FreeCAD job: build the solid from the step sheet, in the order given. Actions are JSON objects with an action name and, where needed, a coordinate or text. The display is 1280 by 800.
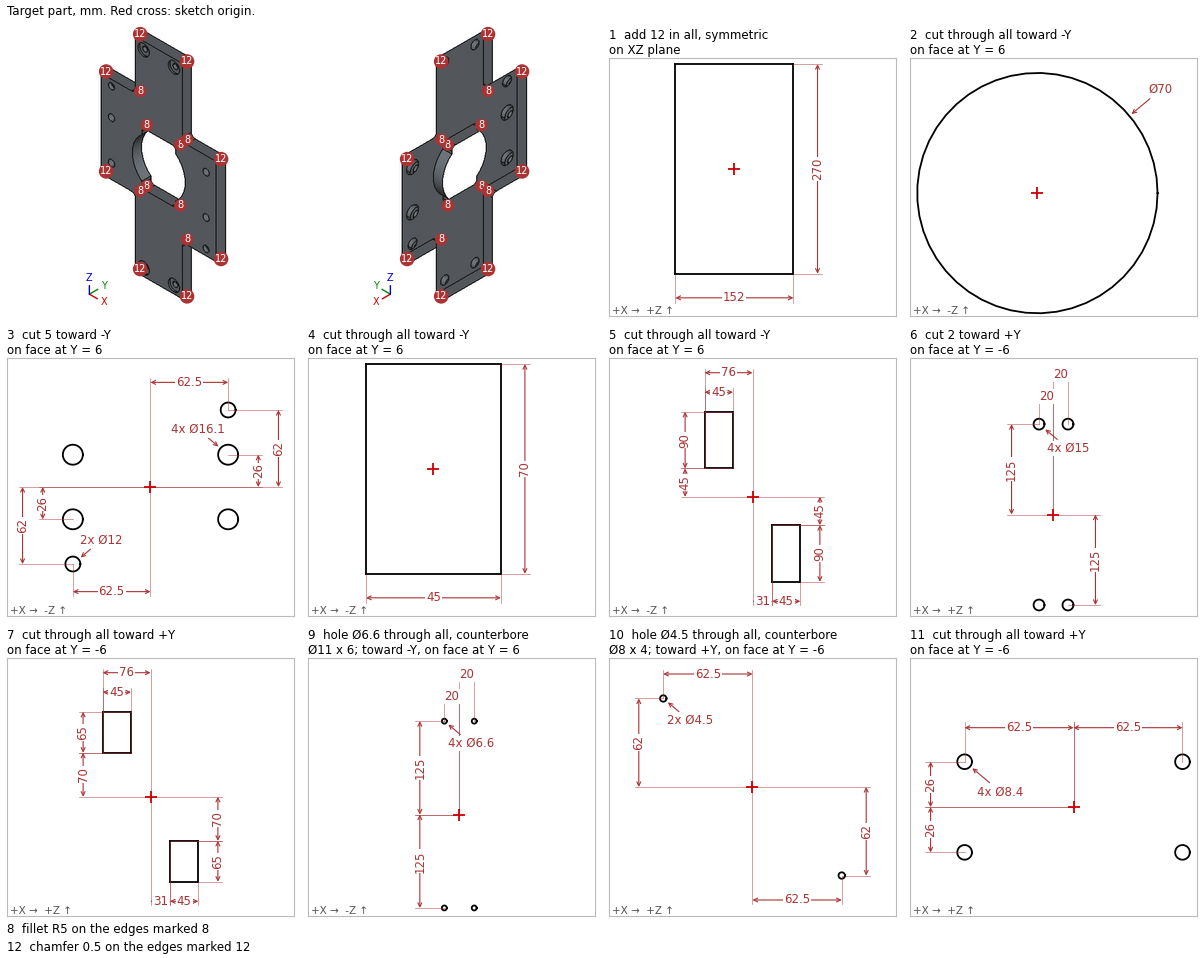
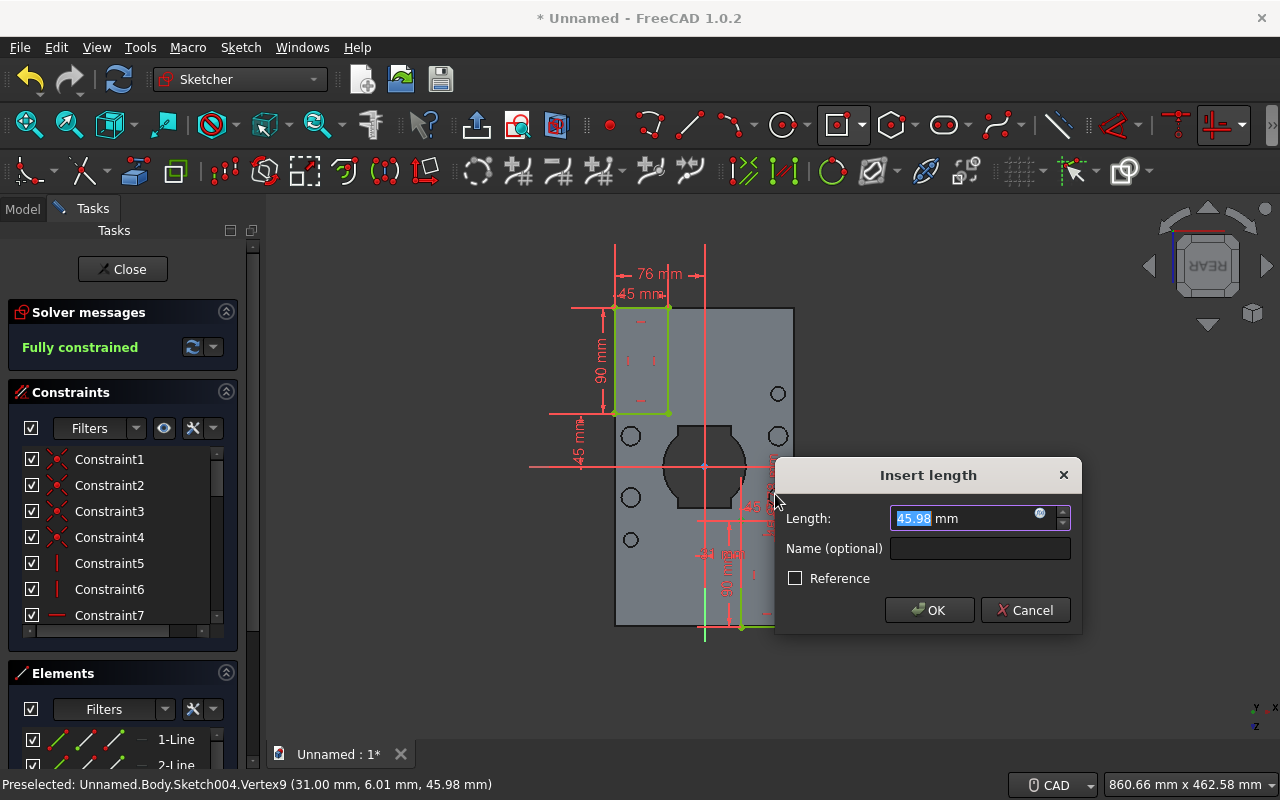
{"action": "type", "text": "45"}
{"action": "key", "text": "Return"}
{"action": "key", "text": "Escape"}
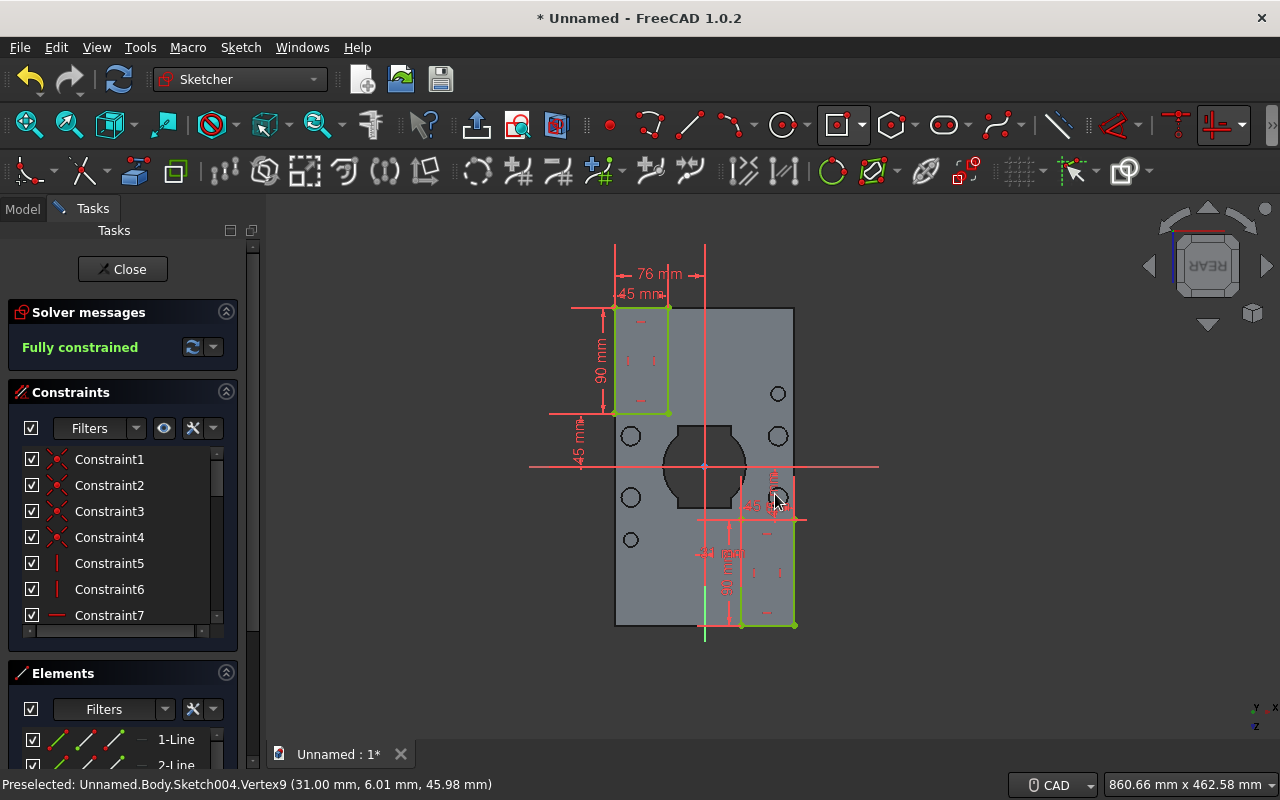
{"action": "left_click", "coordinate": [123, 269]}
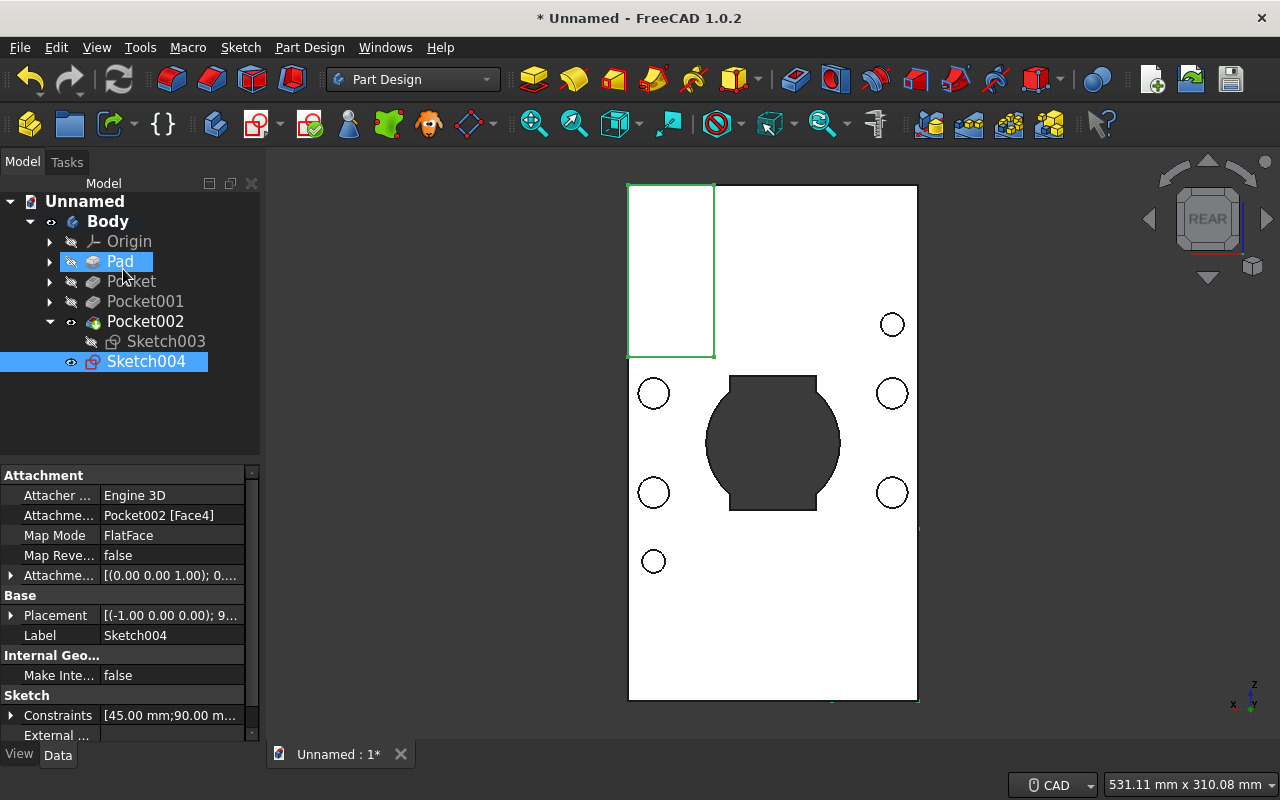
{"action": "left_click", "coordinate": [796, 80]}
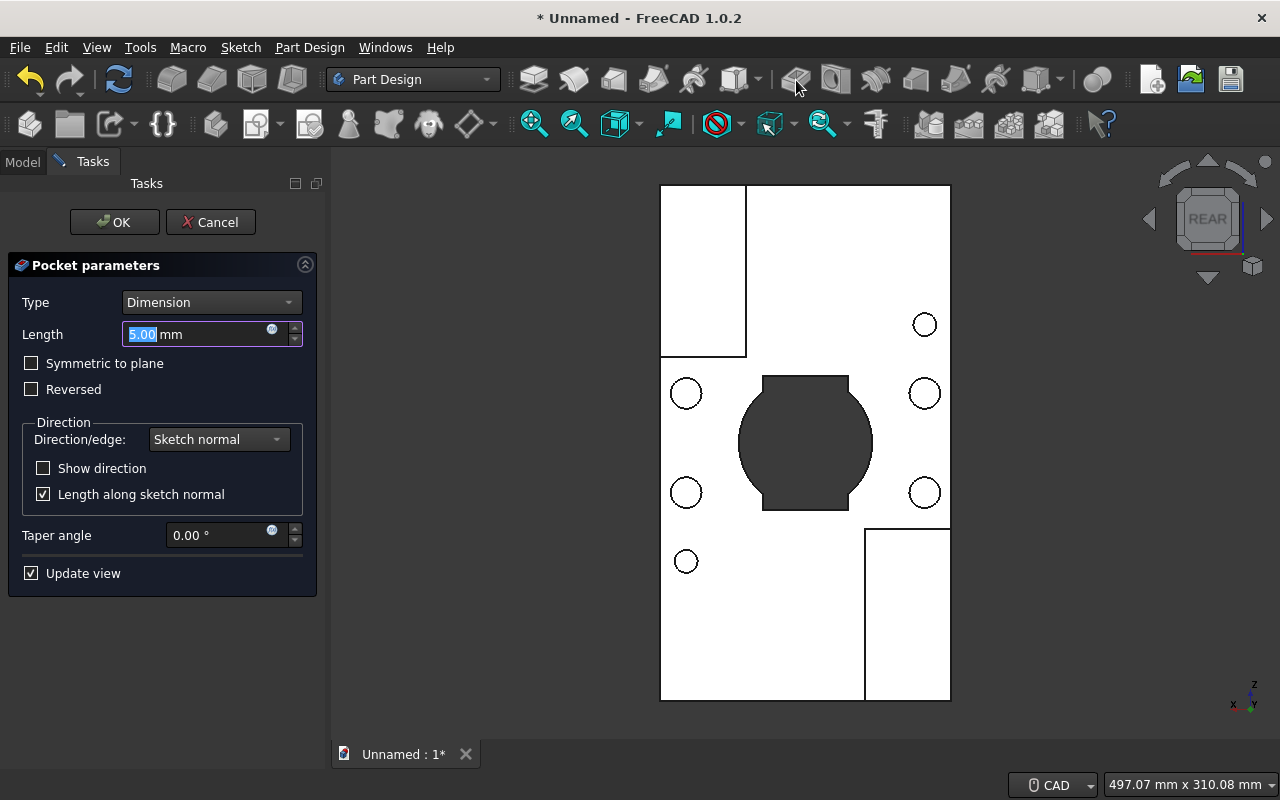
{"action": "left_click", "coordinate": [212, 302]}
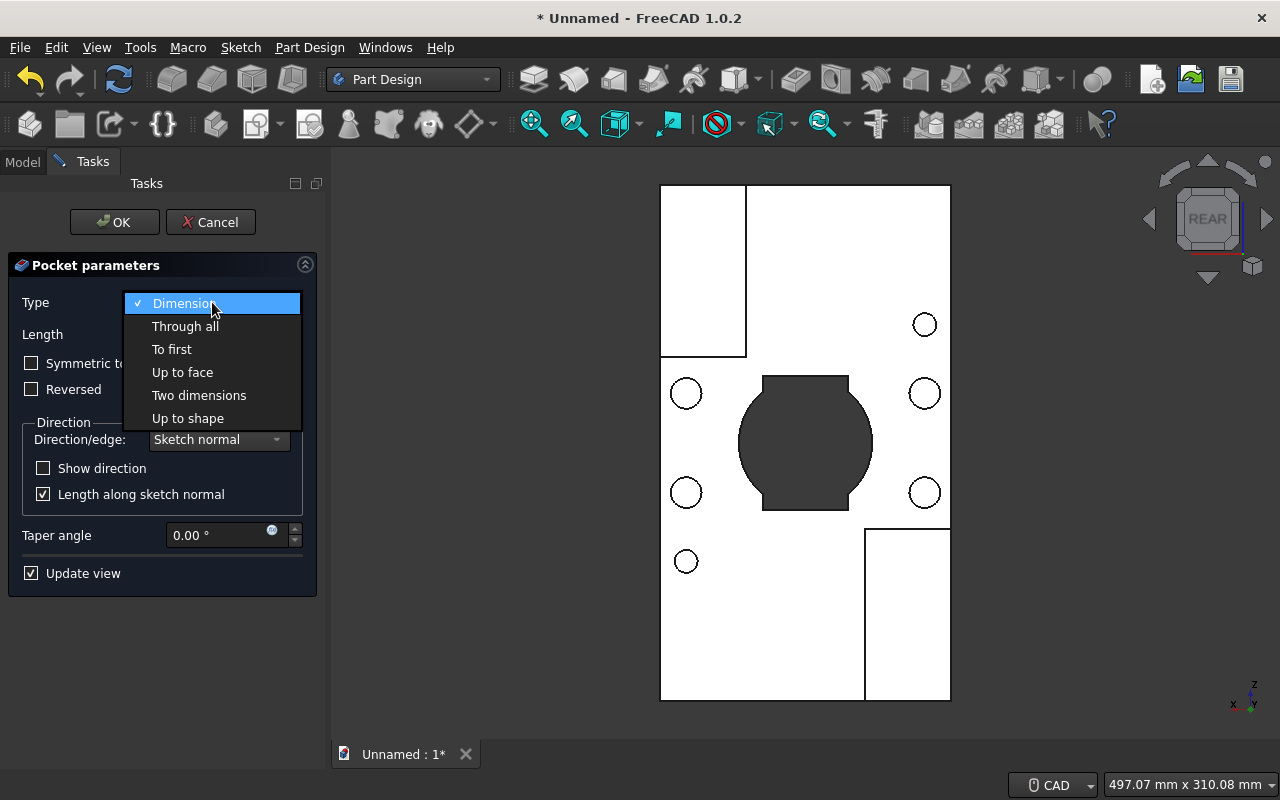
{"action": "left_click", "coordinate": [212, 326]}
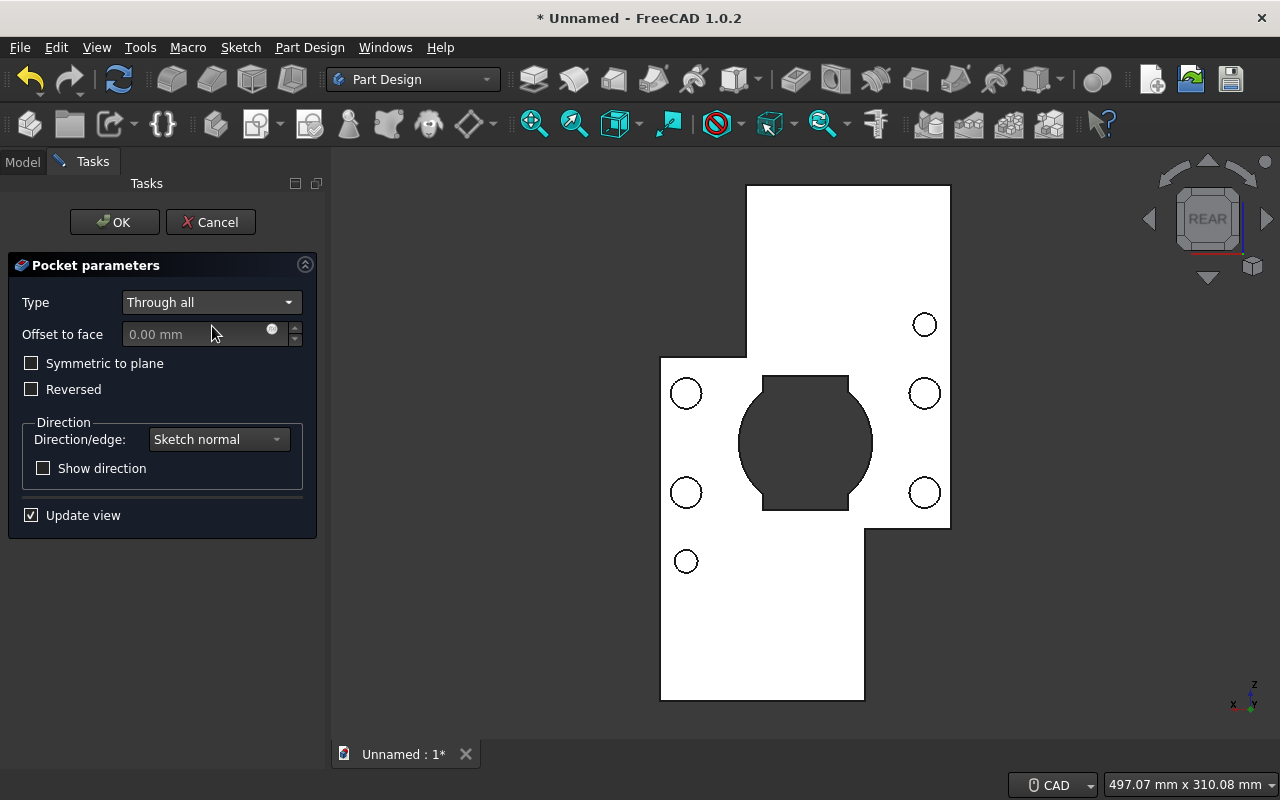
{"action": "left_click", "coordinate": [115, 222]}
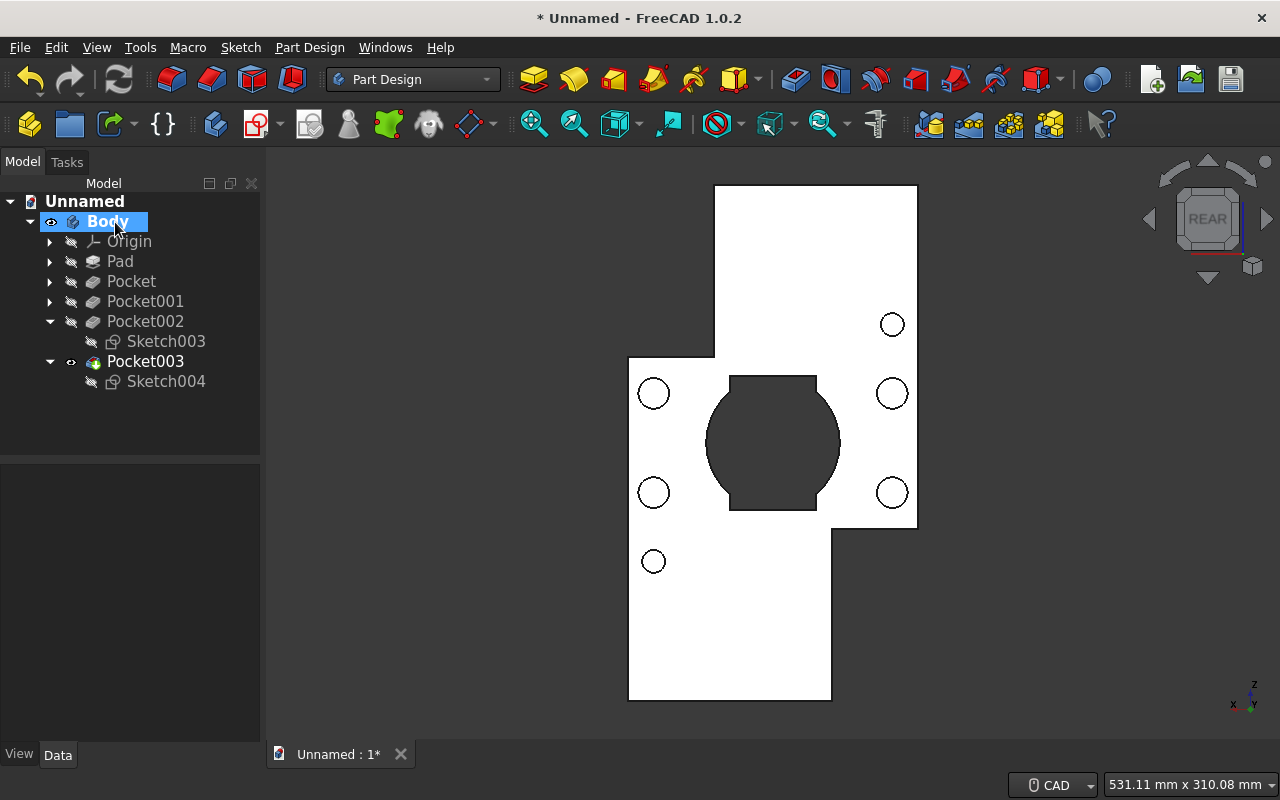
{"action": "key", "text": "0"}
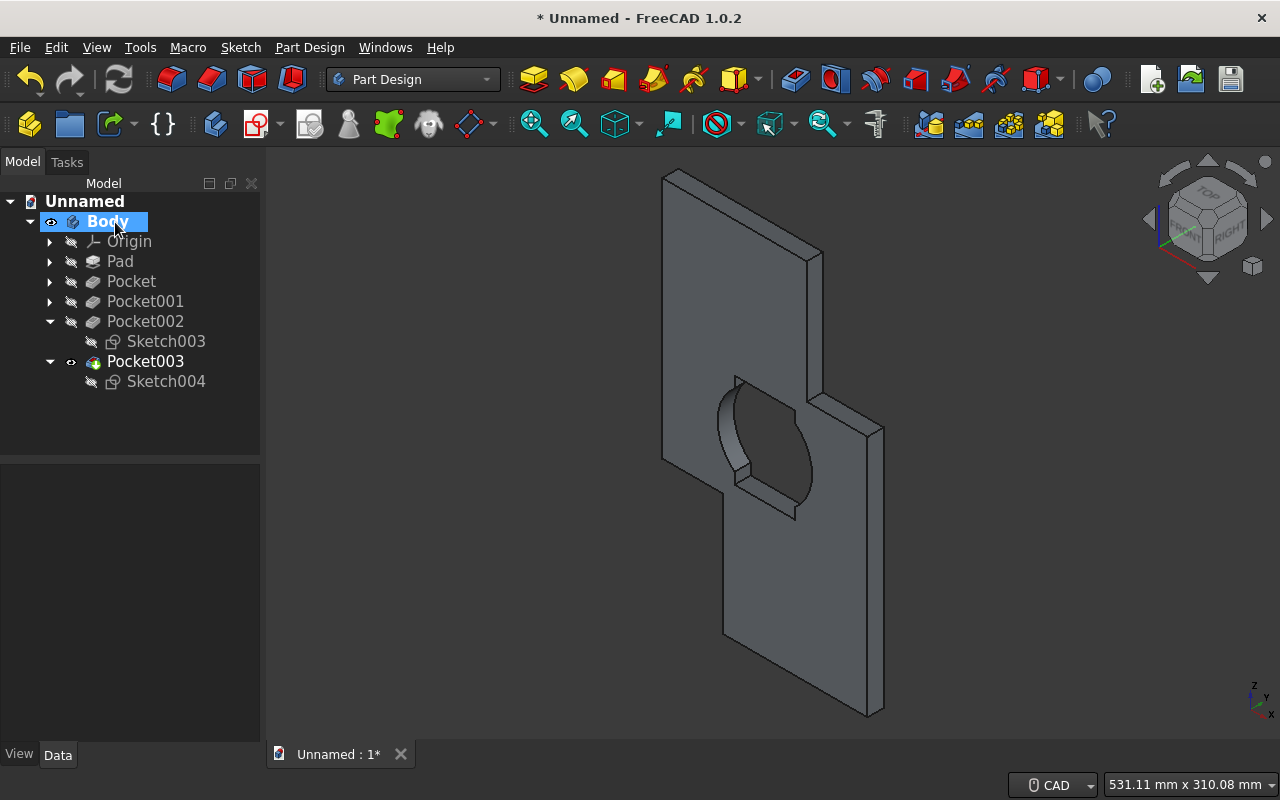
{"action": "left_click", "coordinate": [794, 584]}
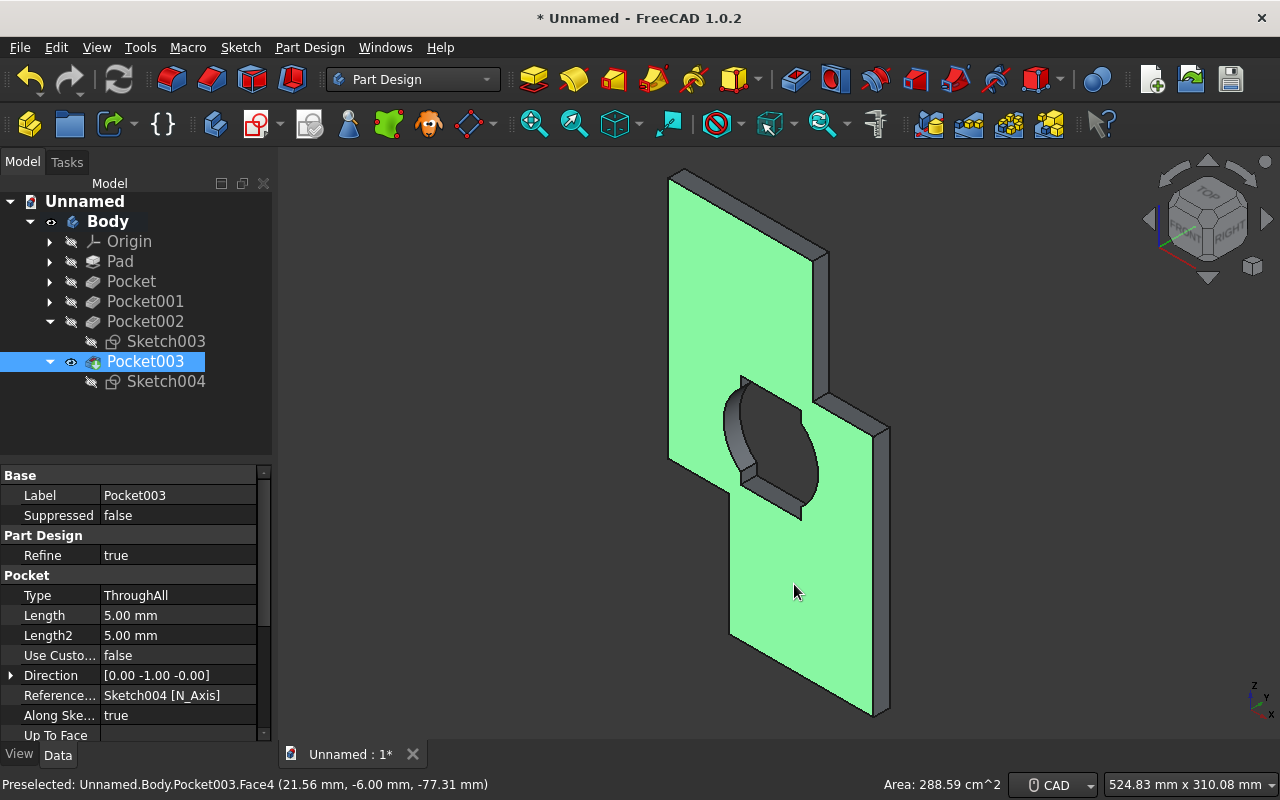
{"action": "left_click", "coordinate": [256, 124]}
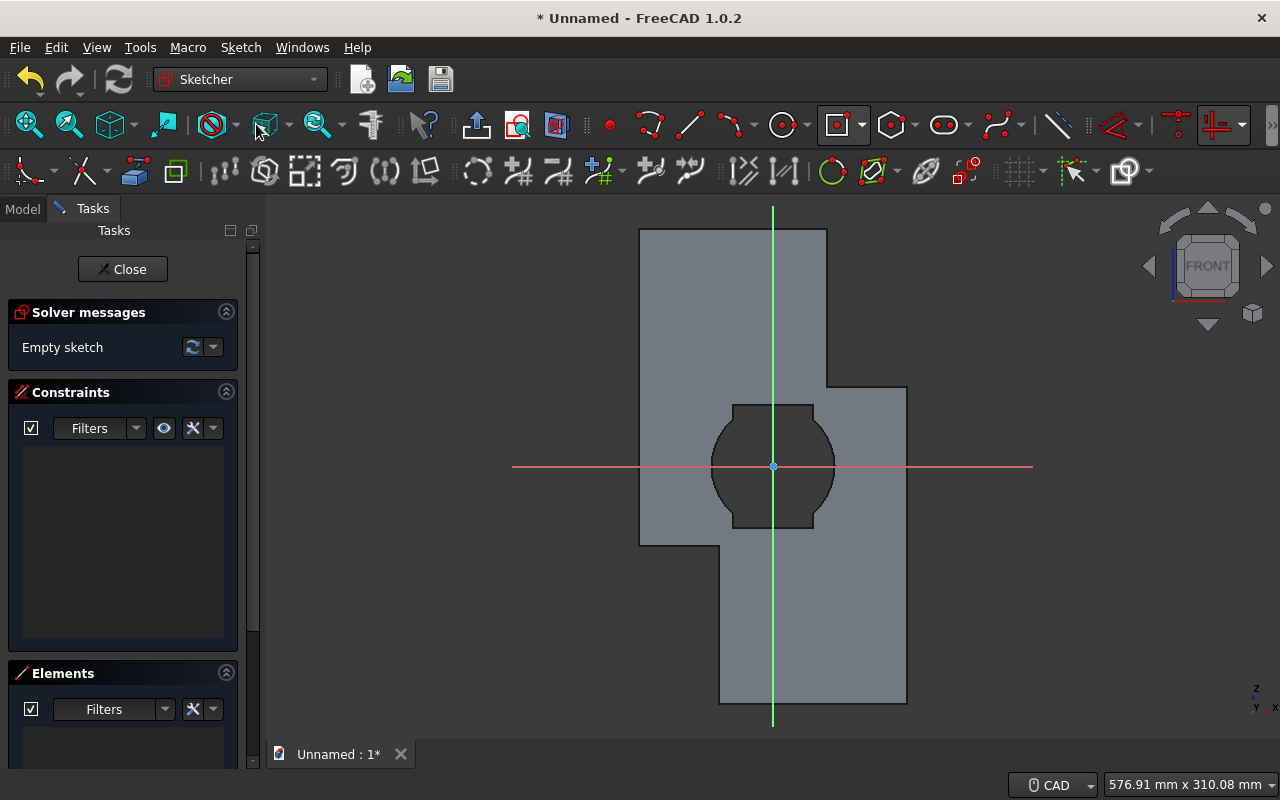
{"action": "scroll", "coordinate": [395, 466], "scroll_direction": "down", "scroll_amount": 1}